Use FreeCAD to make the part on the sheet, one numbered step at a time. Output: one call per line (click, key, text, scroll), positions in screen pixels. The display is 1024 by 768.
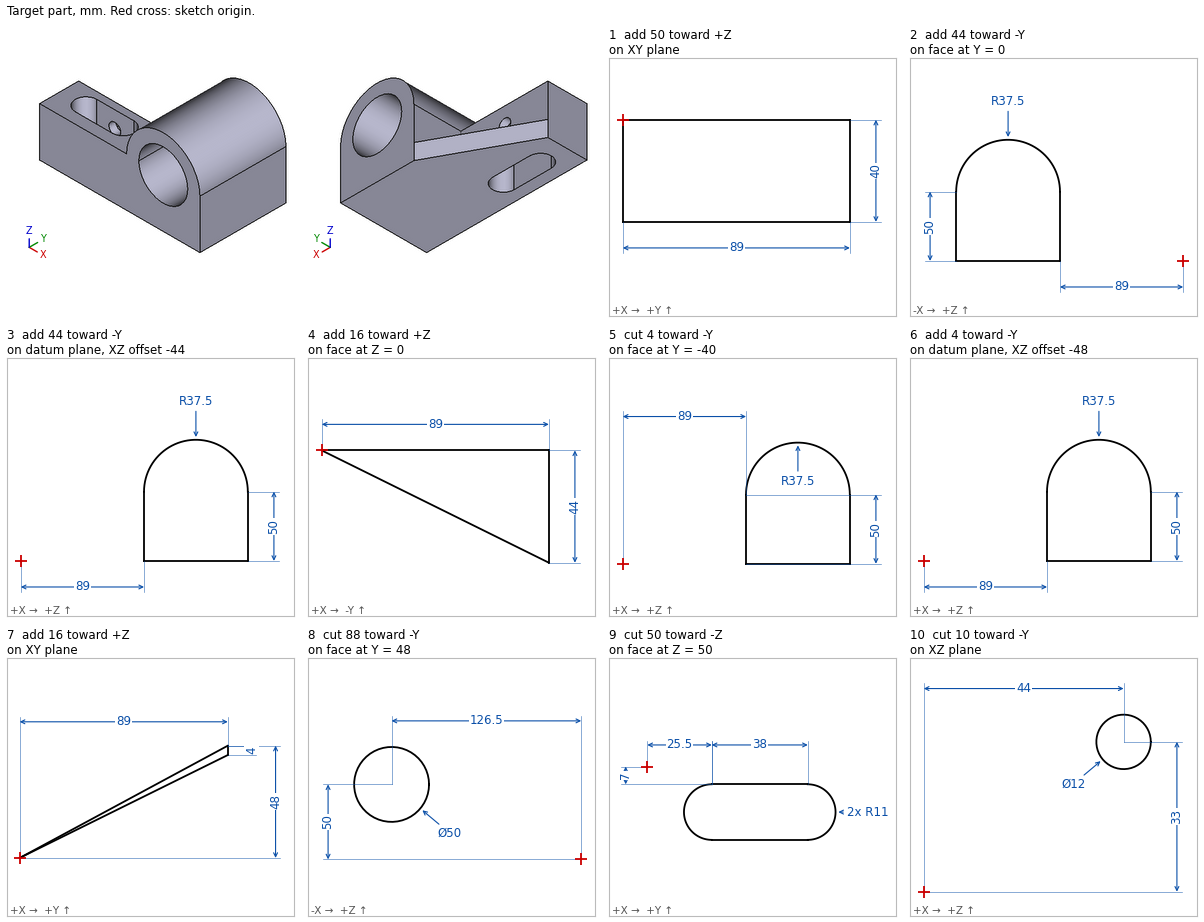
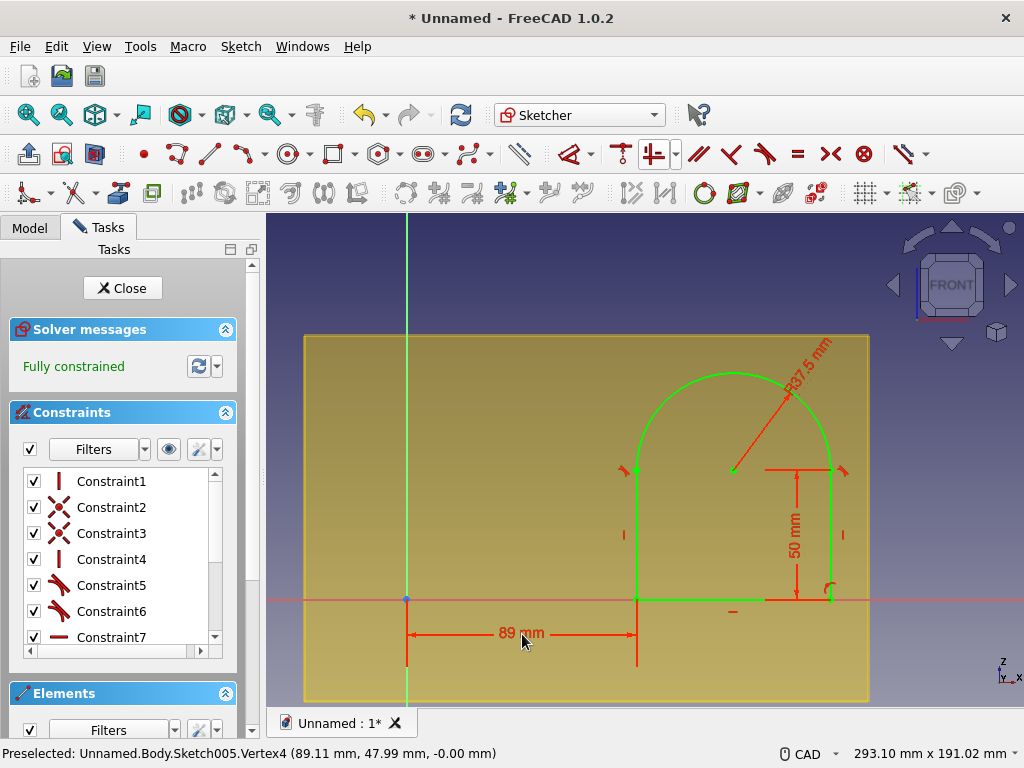
click(123, 288)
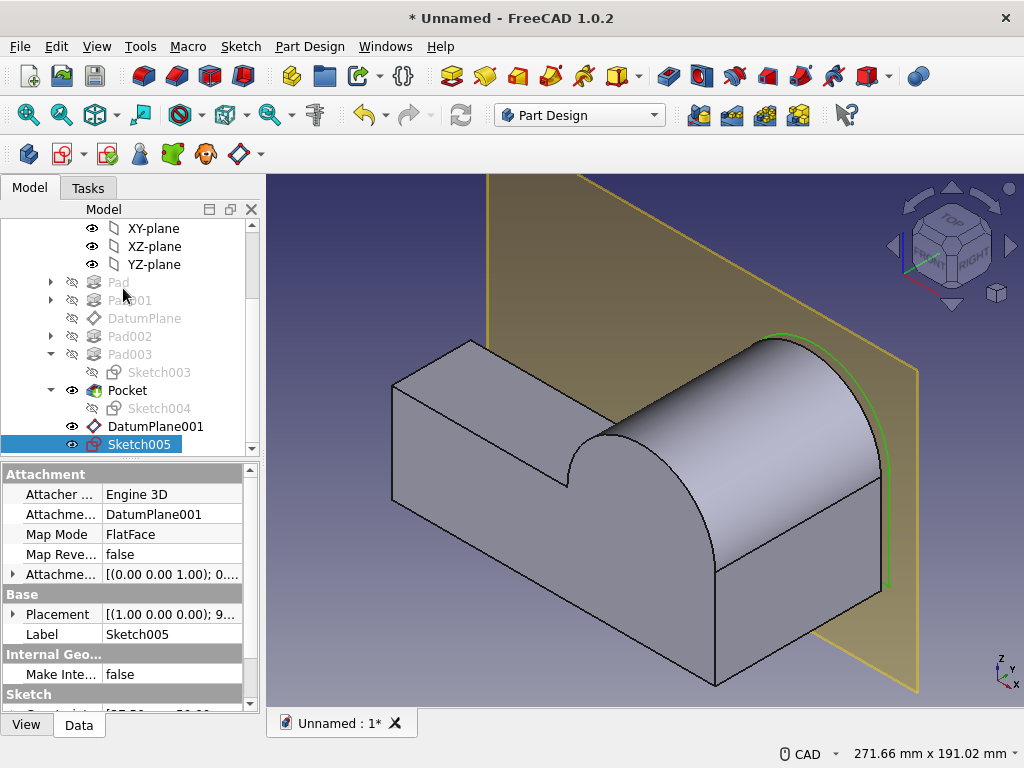
click(452, 76)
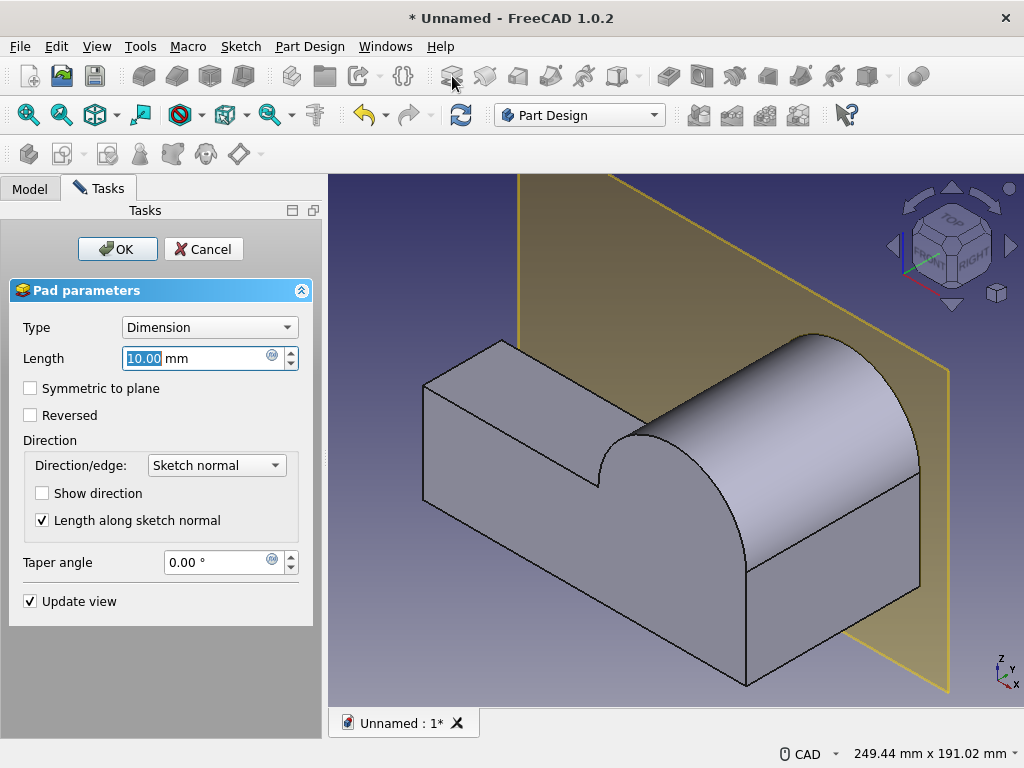
text(4)
key(Tab)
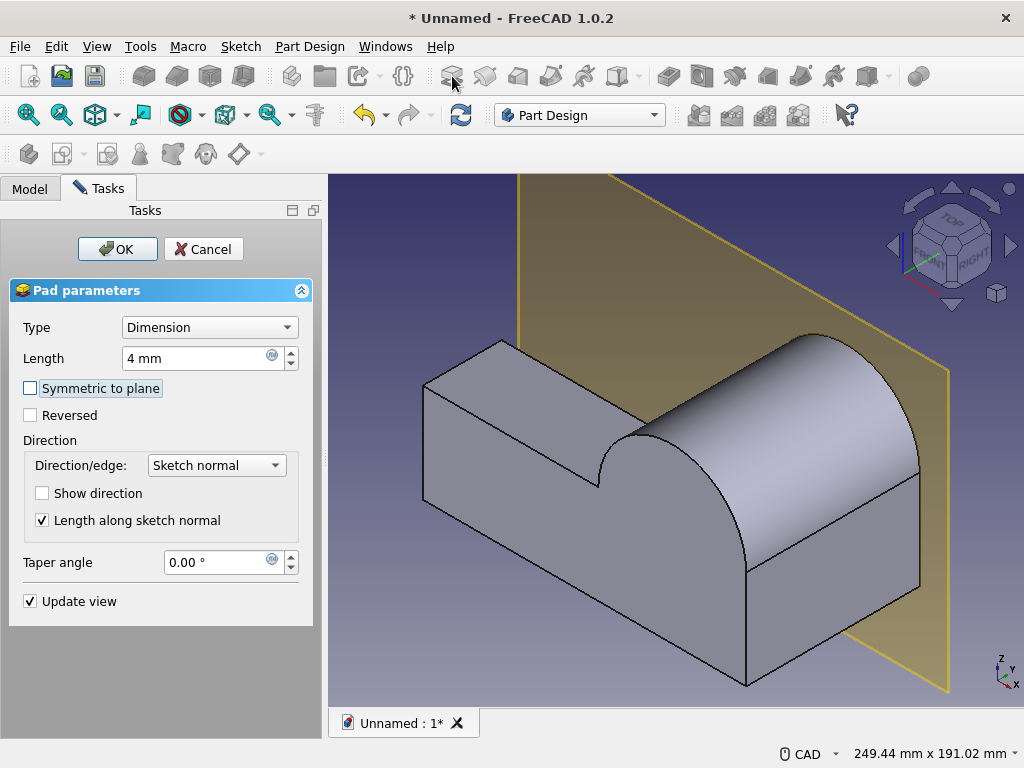
click(118, 249)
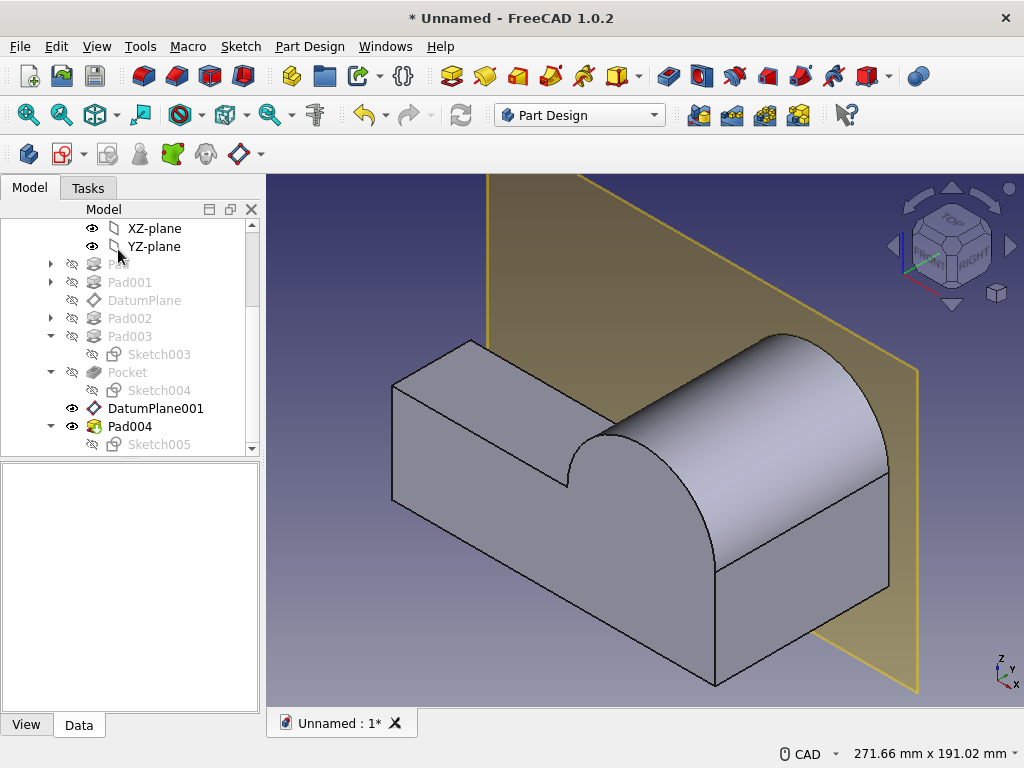
click(117, 408)
key(space)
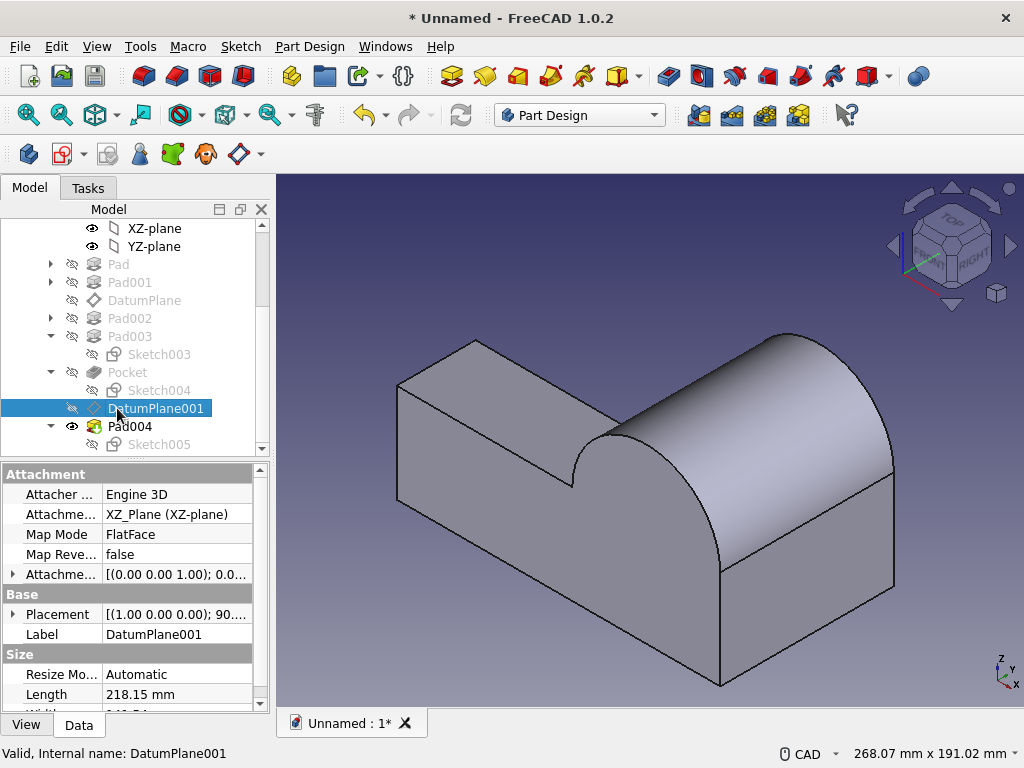
click(316, 667)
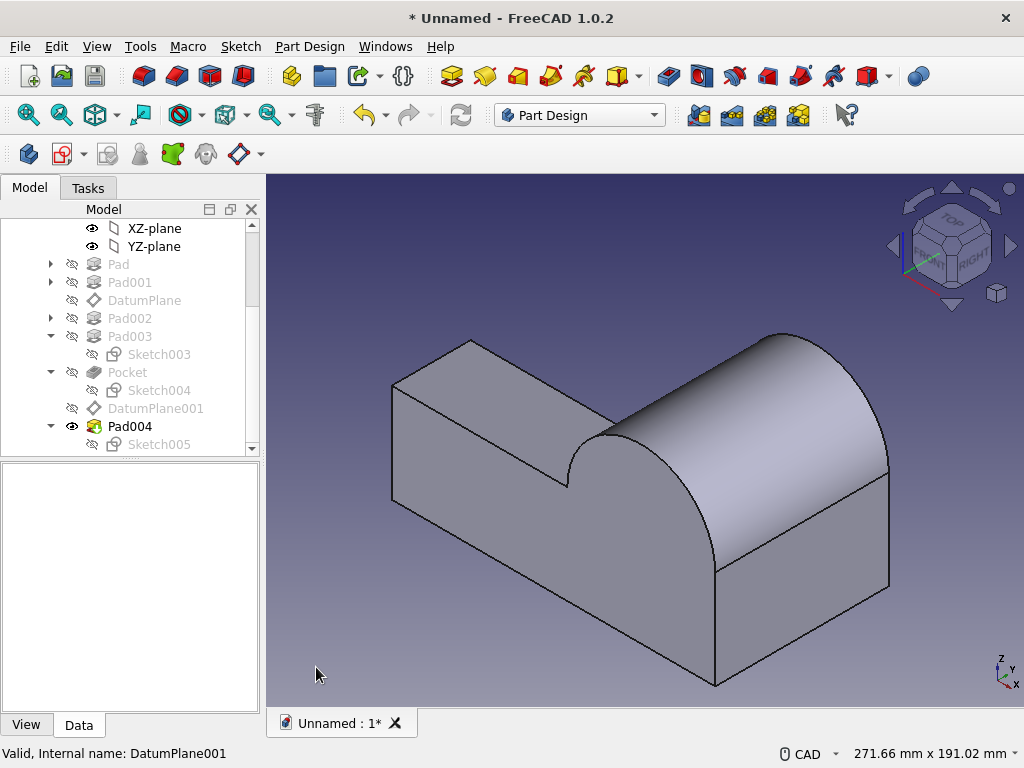
click(62, 154)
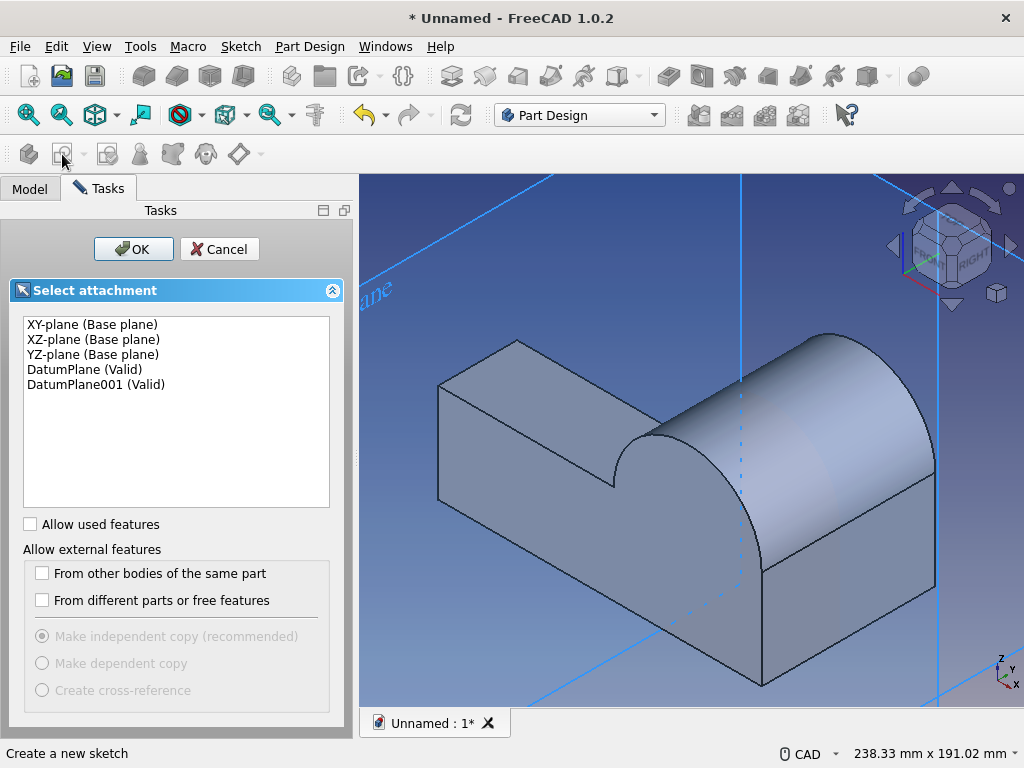
click(84, 324)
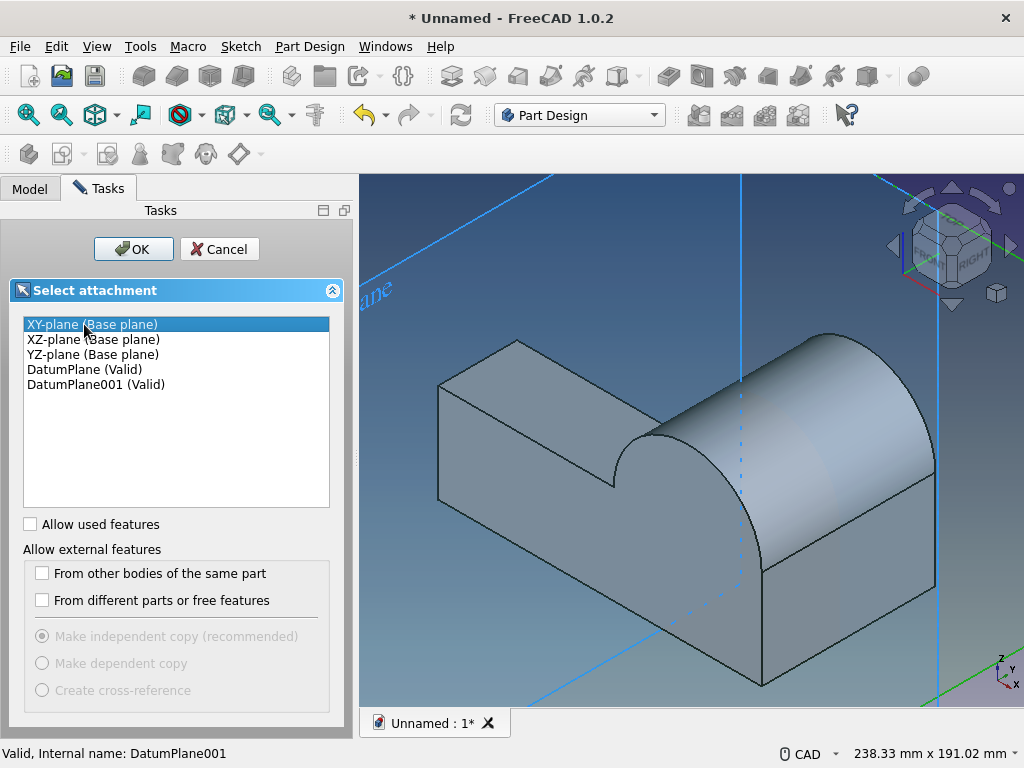
click(134, 249)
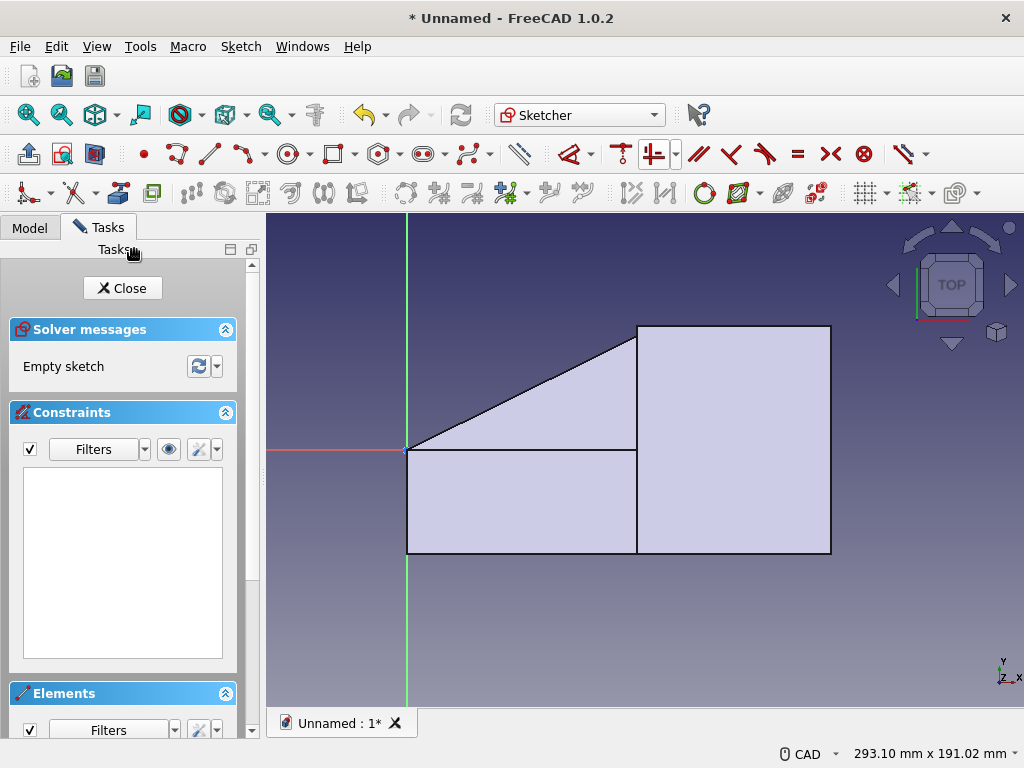
click(95, 154)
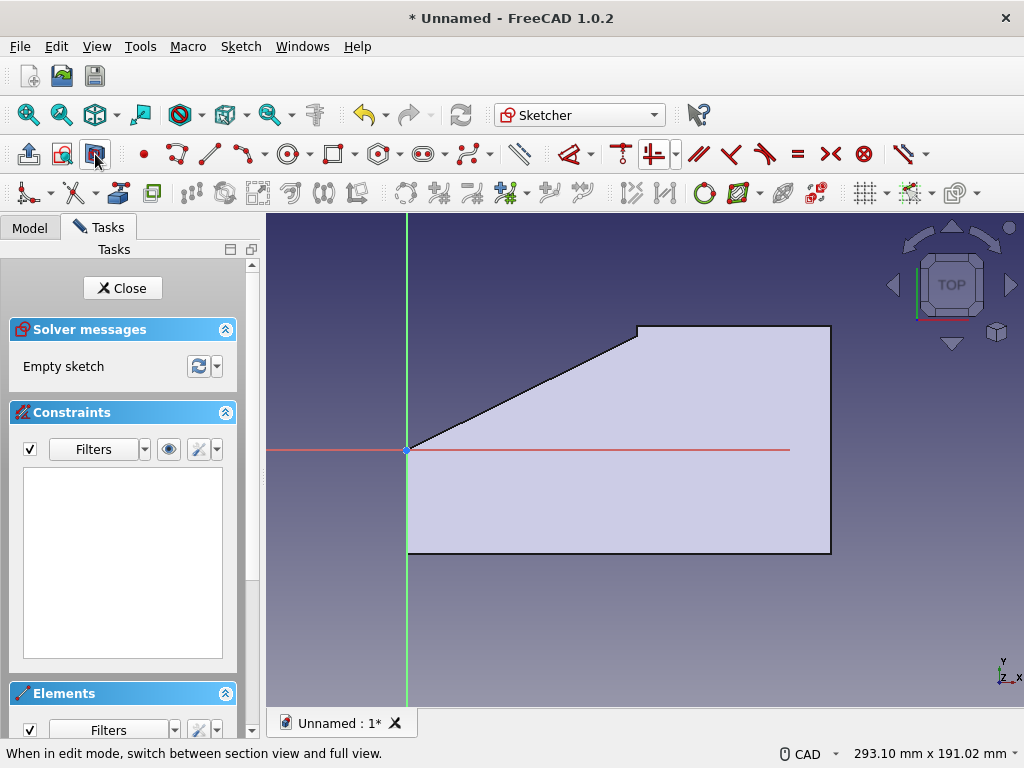
scroll(455, 301, up, 3)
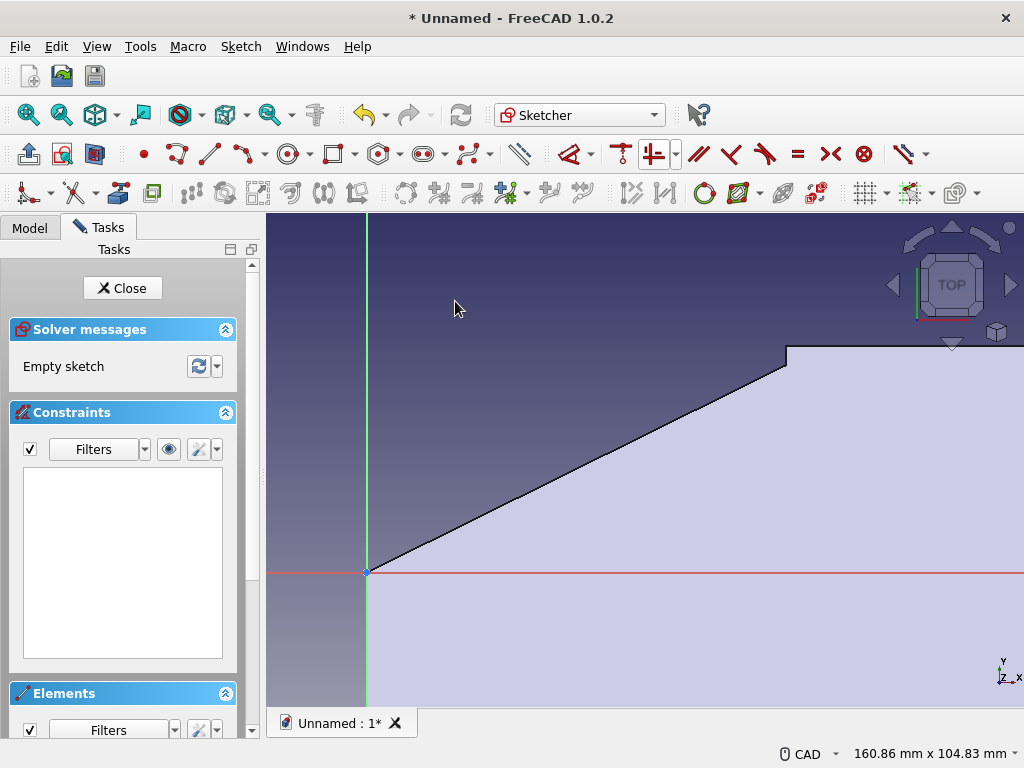
click(177, 154)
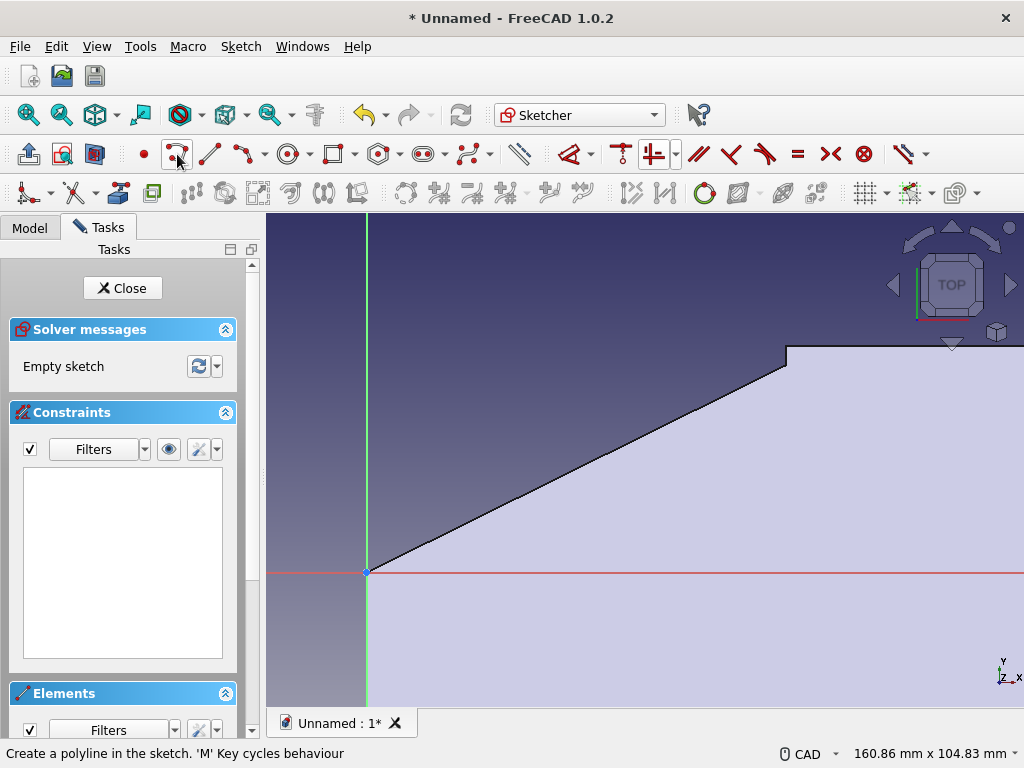
click(367, 573)
click(786, 346)
click(786, 365)
click(367, 573)
key(Escape)
key(Escape)